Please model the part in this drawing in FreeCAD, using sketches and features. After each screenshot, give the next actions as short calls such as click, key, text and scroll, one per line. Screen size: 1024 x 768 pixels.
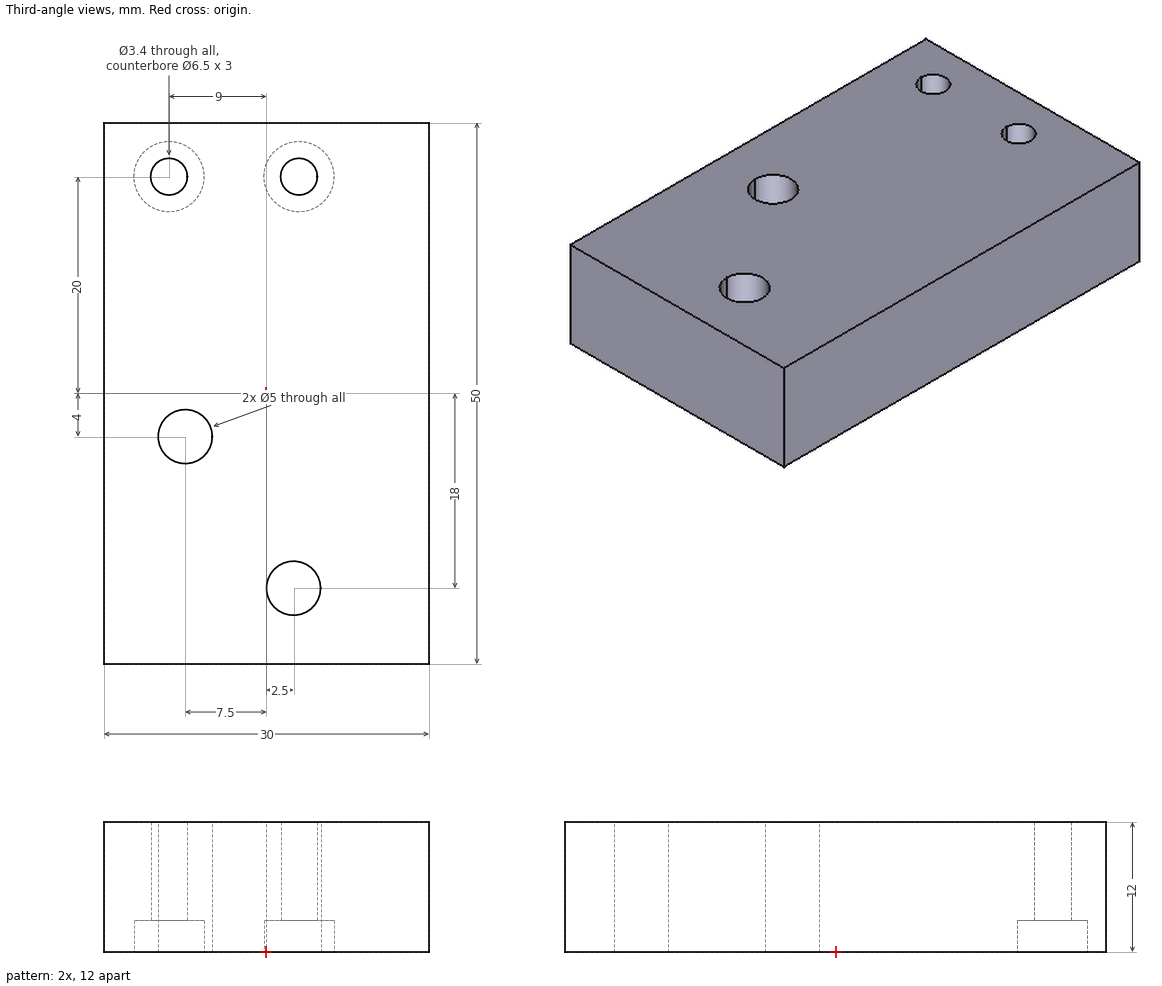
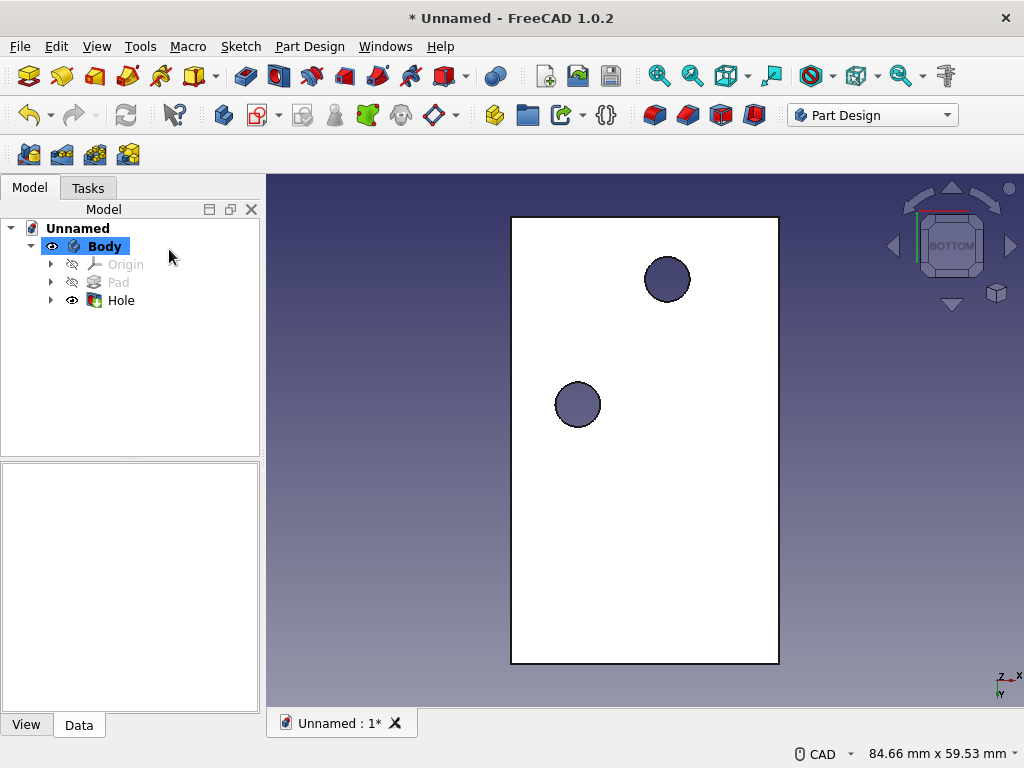
click(645, 503)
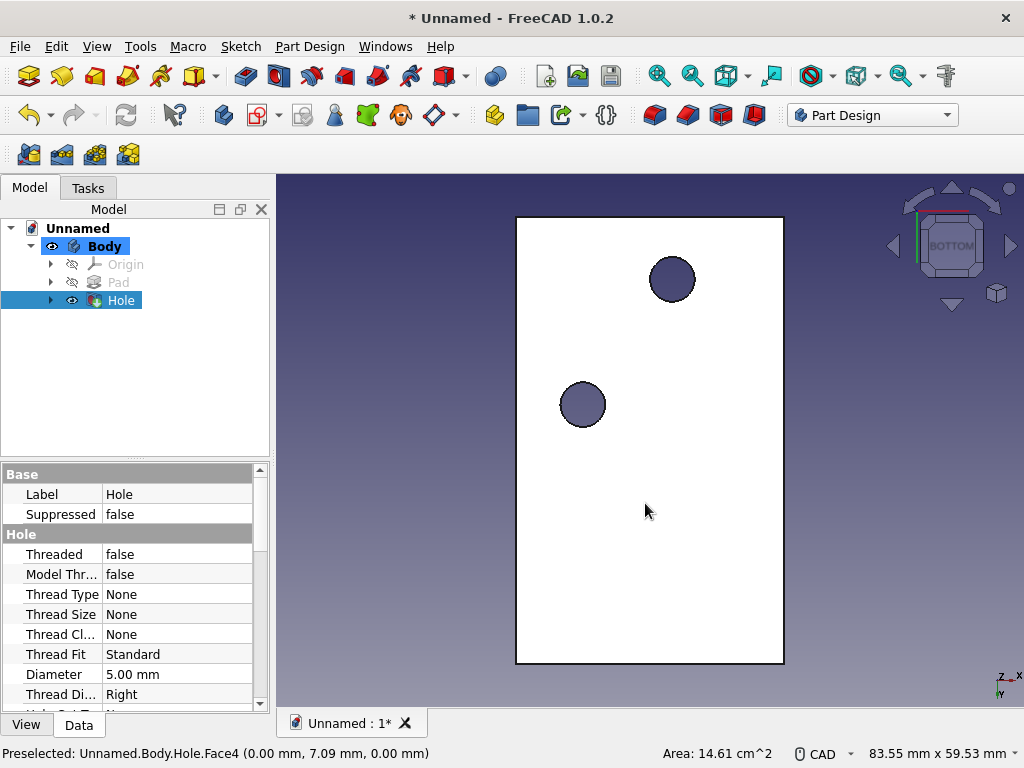
click(256, 116)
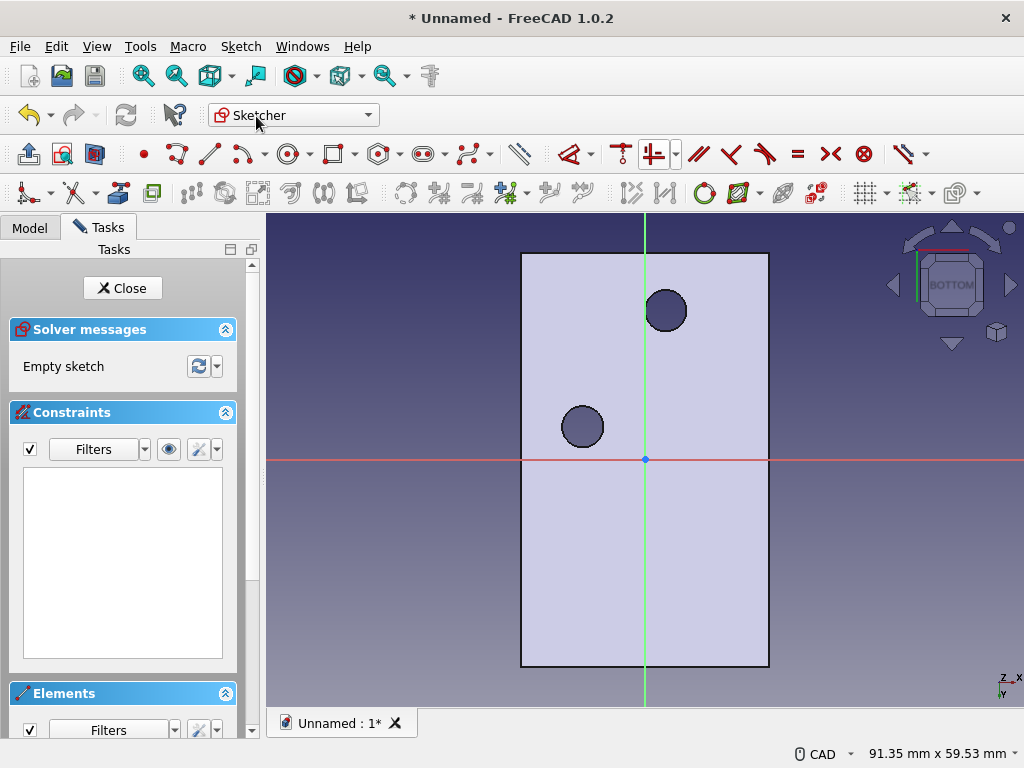
scroll(570, 643, up, 12)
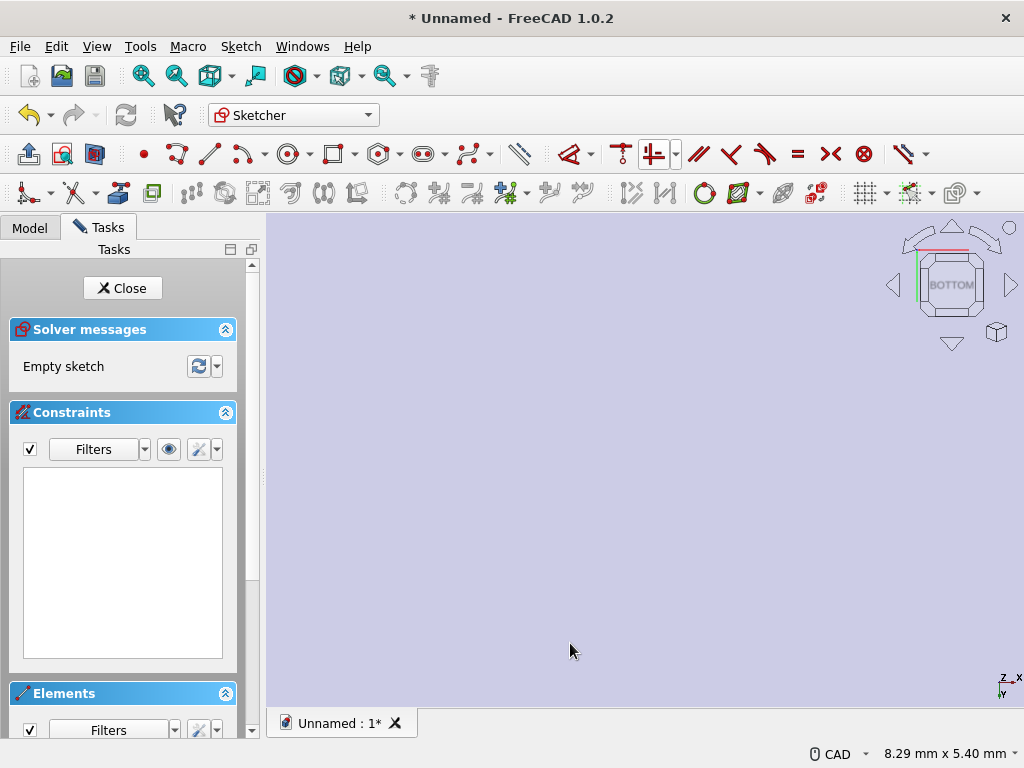
key(g)
key(c)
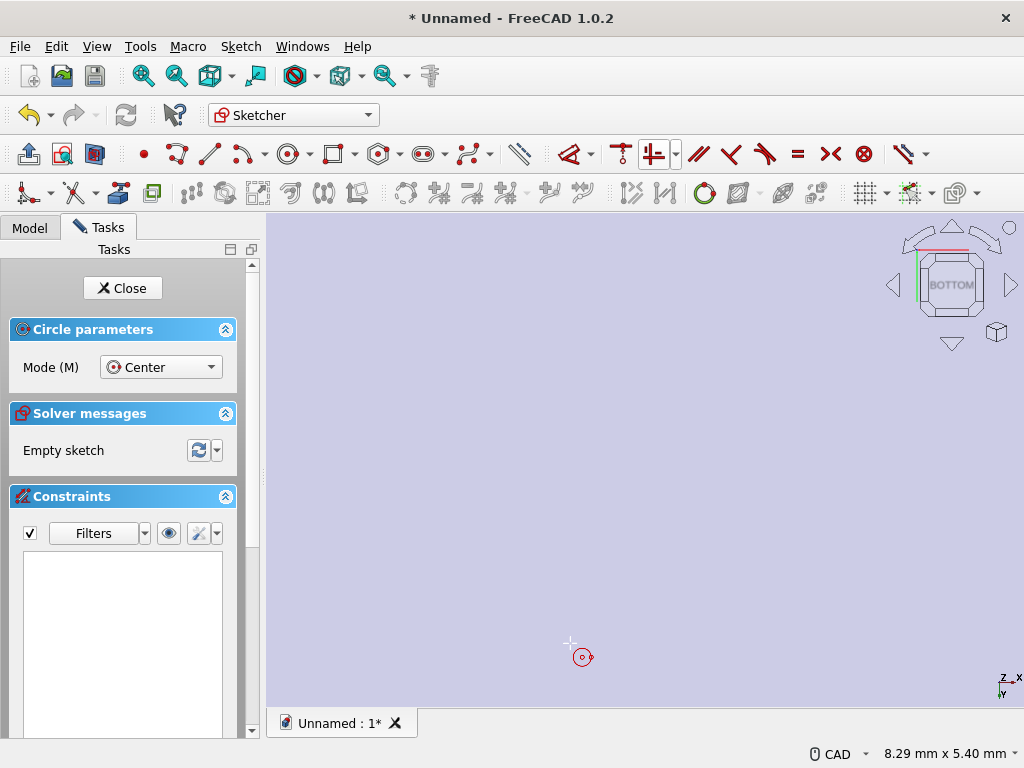
click(569, 446)
move(679, 336)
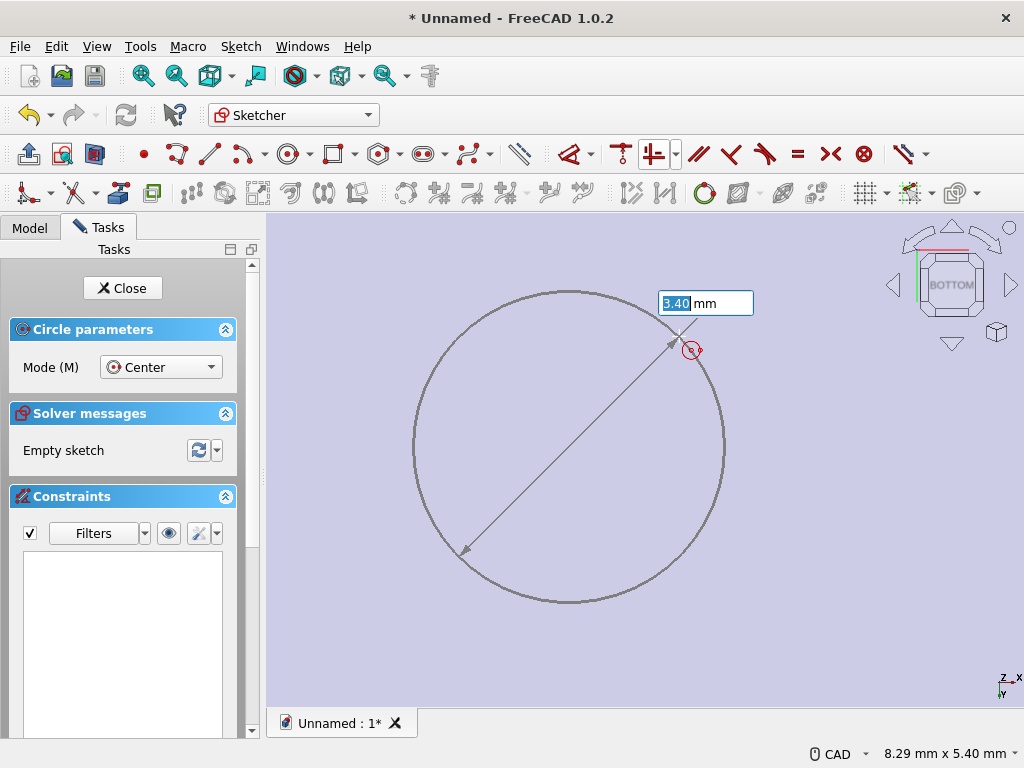
text(3.4)
key(Return)
key(Escape)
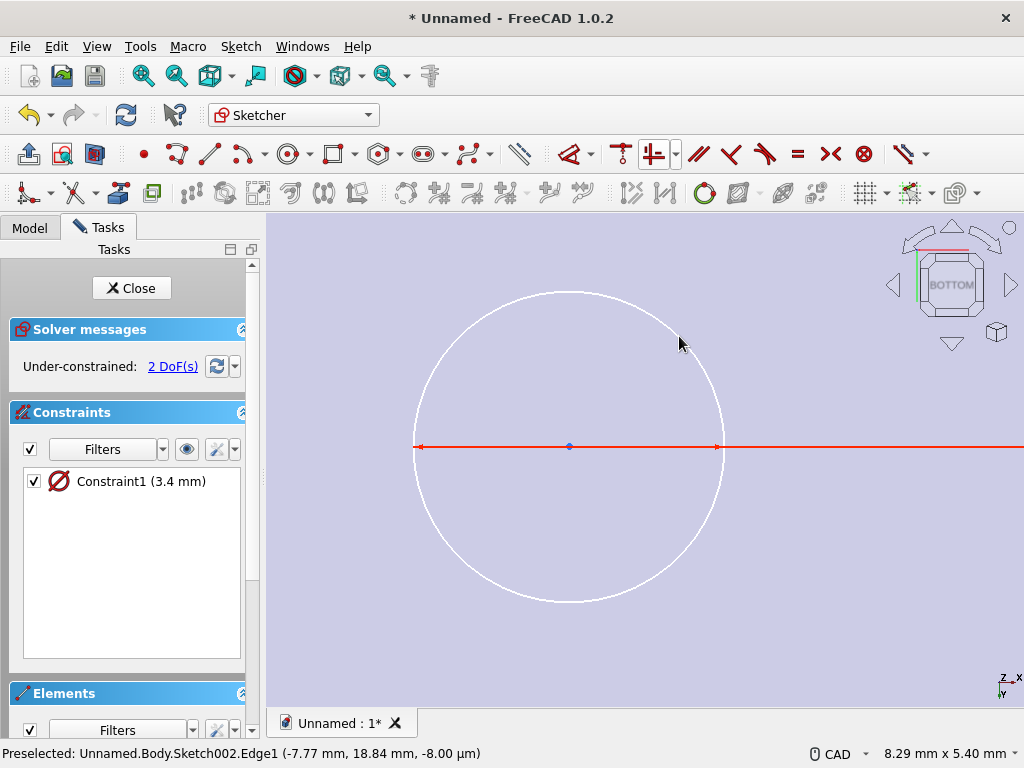
key(d)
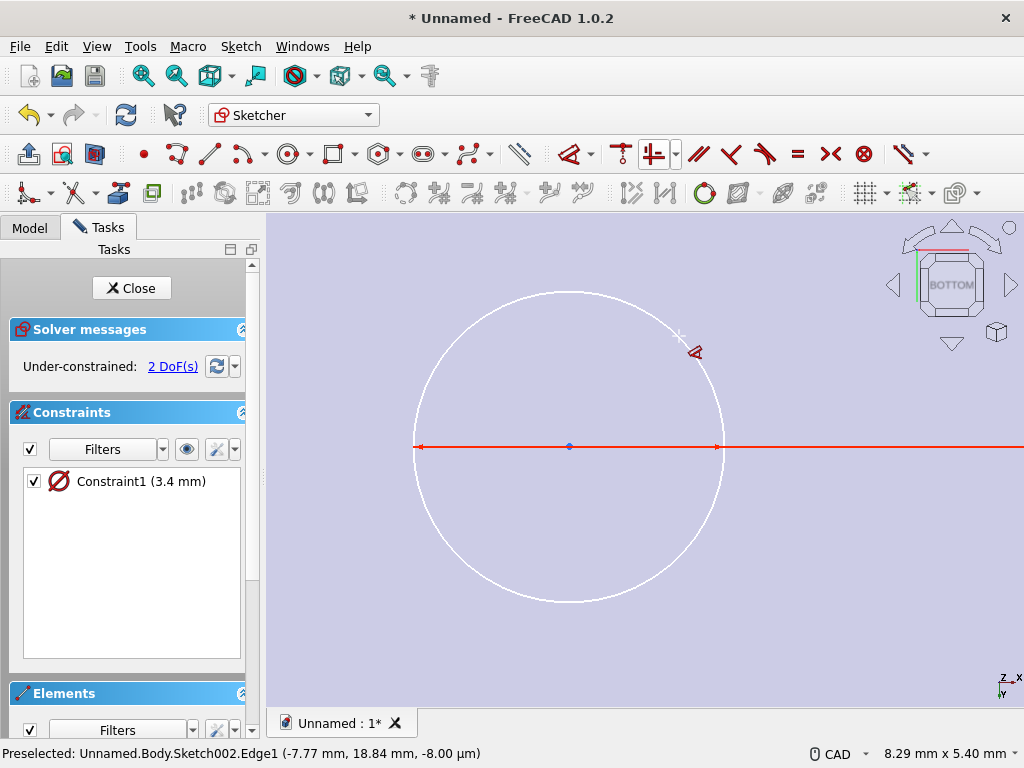
click(569, 447)
click(647, 481)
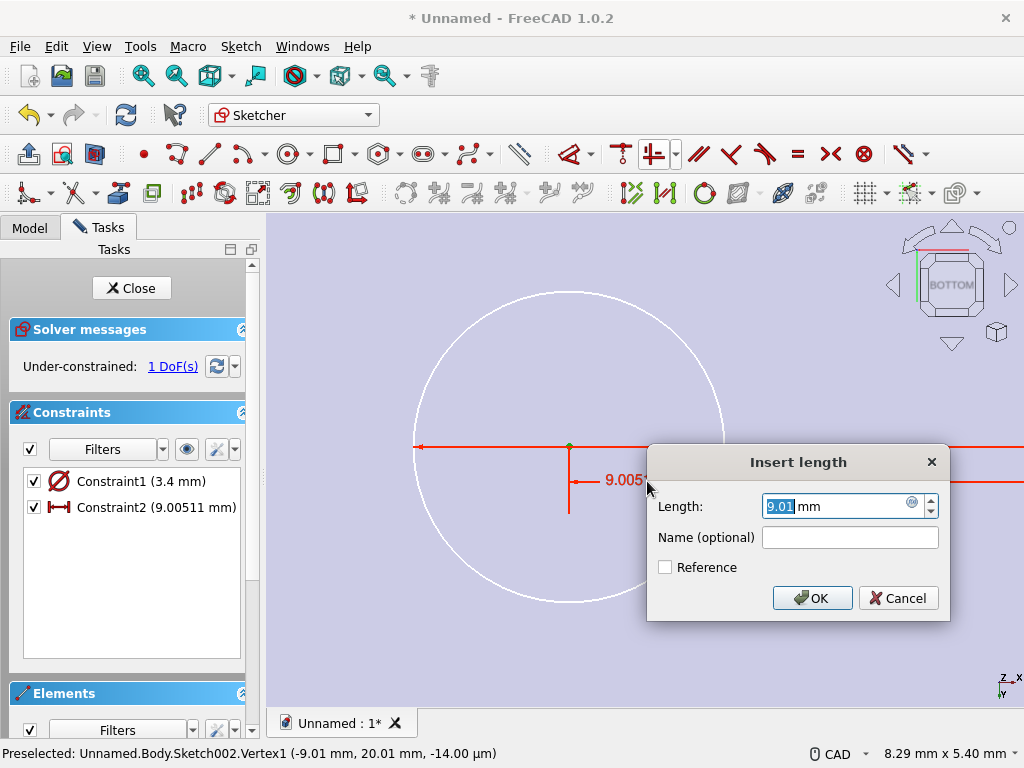
text(9)
key(Return)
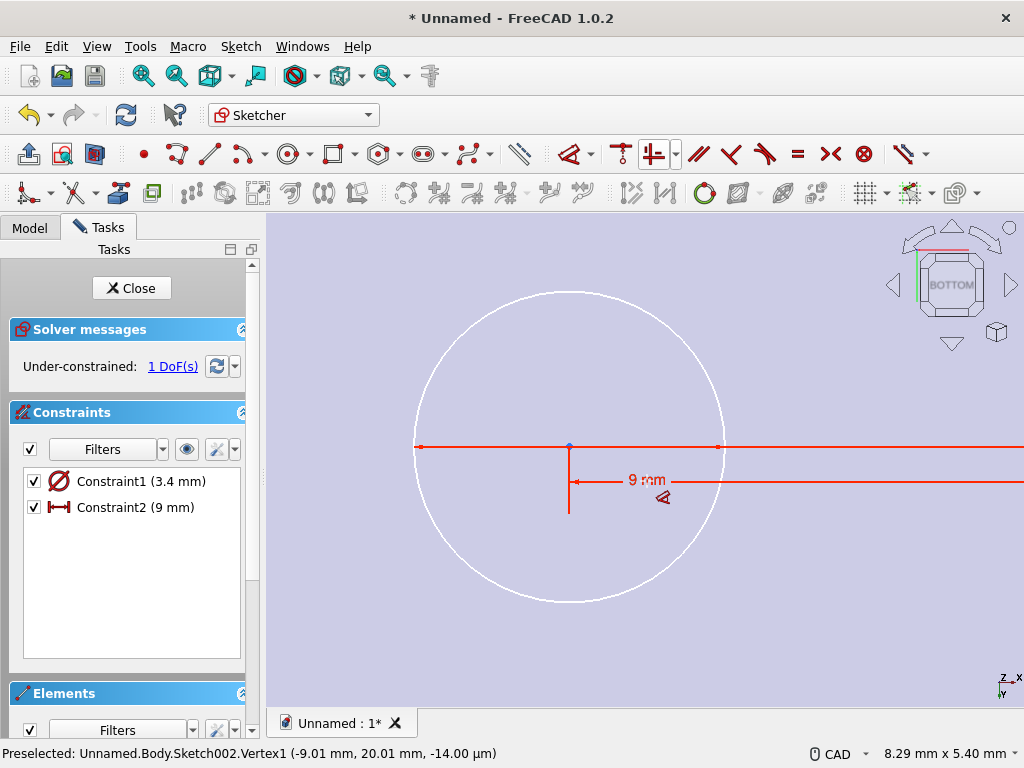
click(569, 447)
click(535, 344)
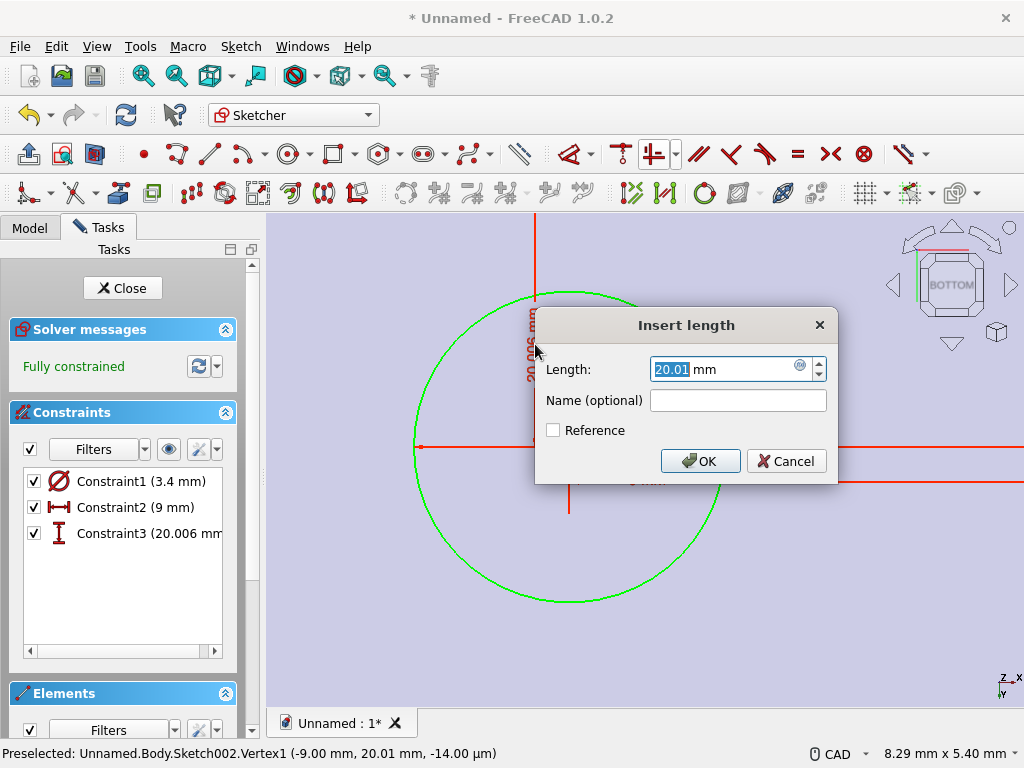
text(20)
key(Return)
key(Escape)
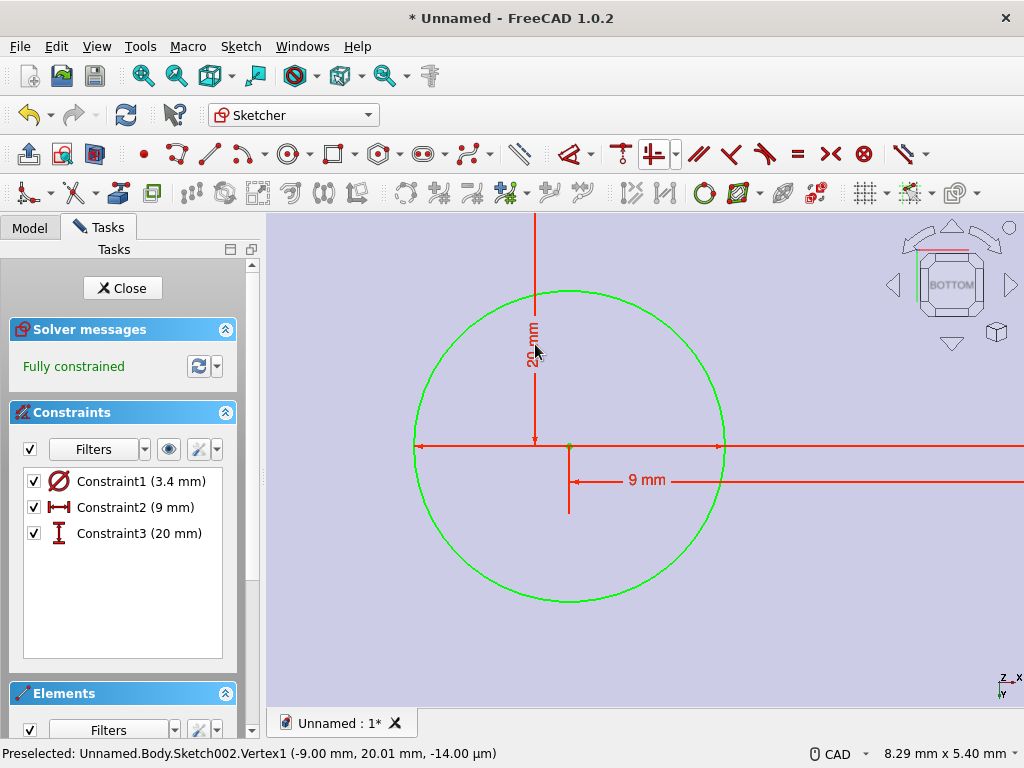
click(123, 288)